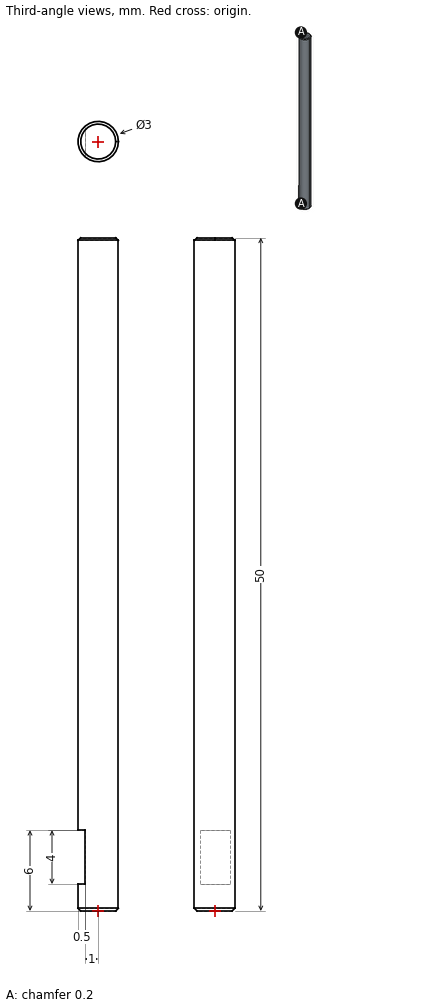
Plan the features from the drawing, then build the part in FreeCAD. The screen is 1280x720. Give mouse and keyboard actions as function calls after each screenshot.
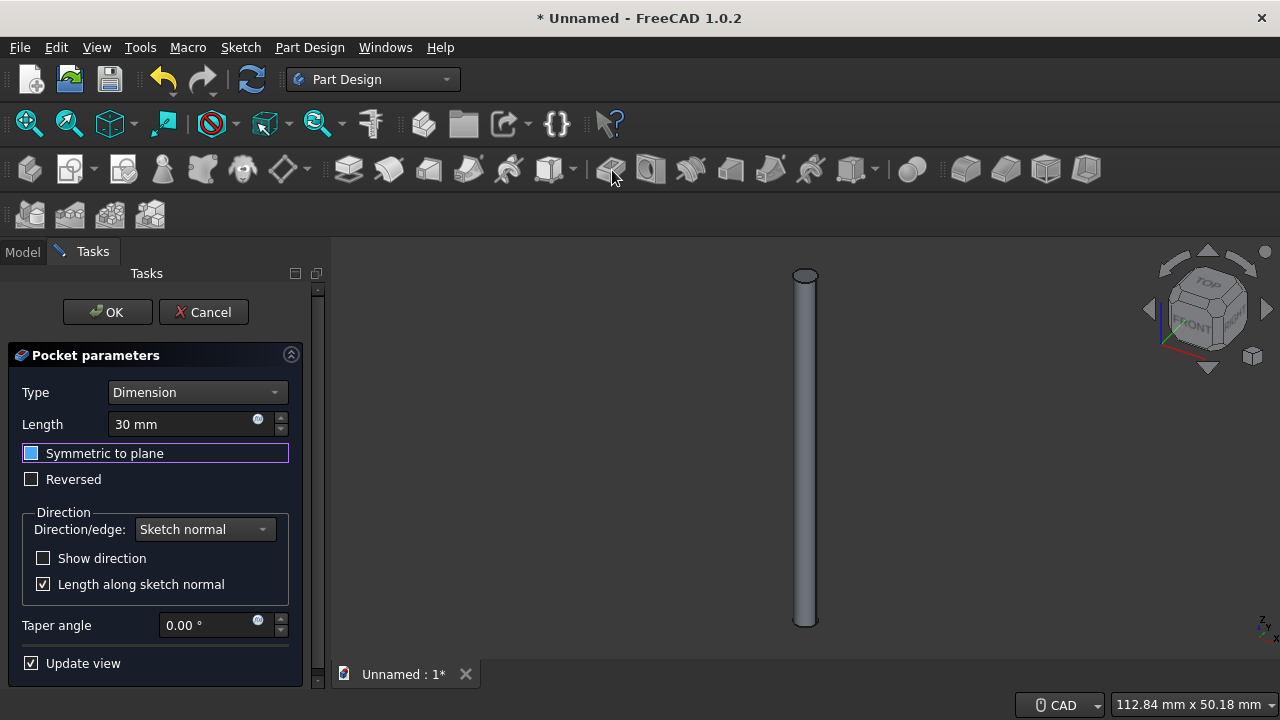
click(30, 453)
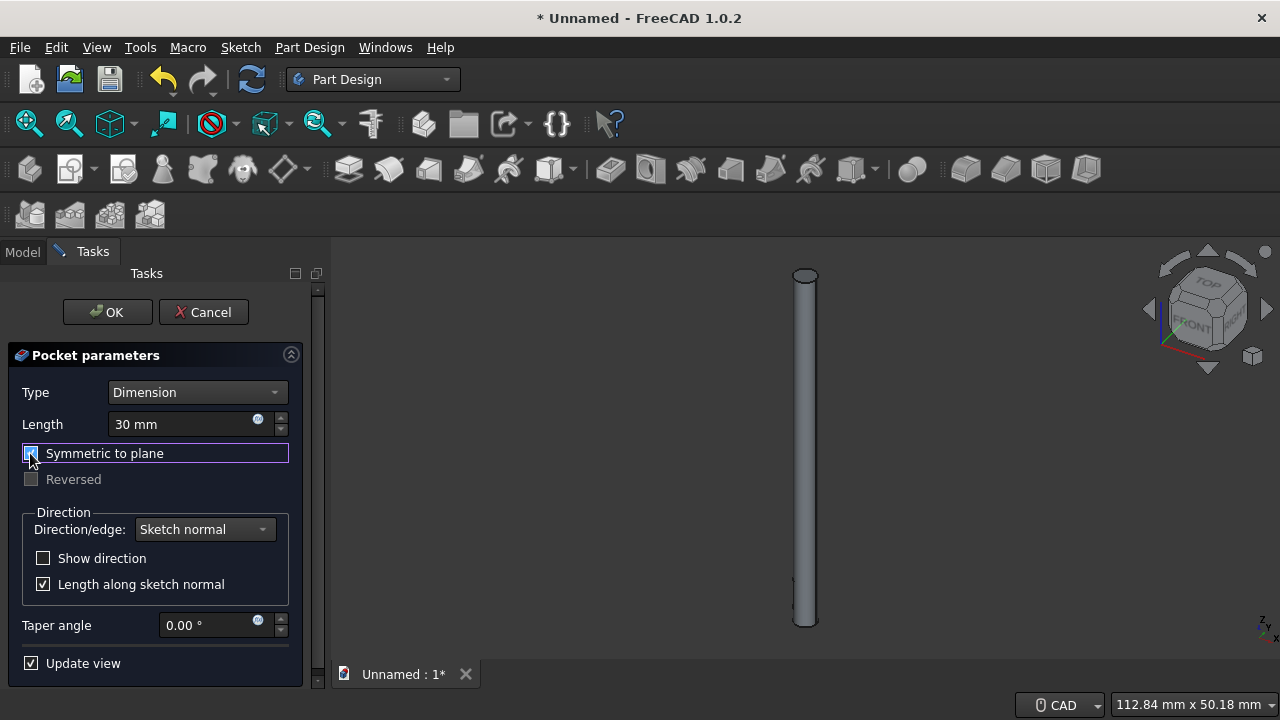
click(108, 312)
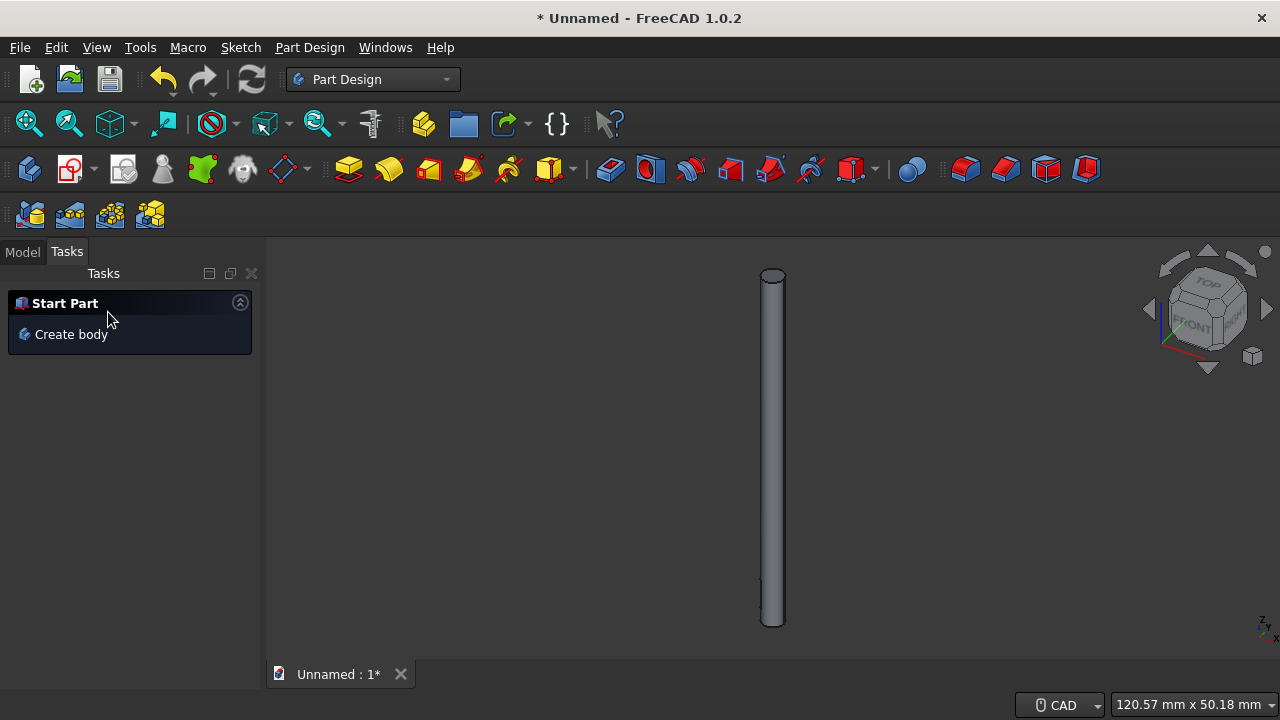
click(764, 624)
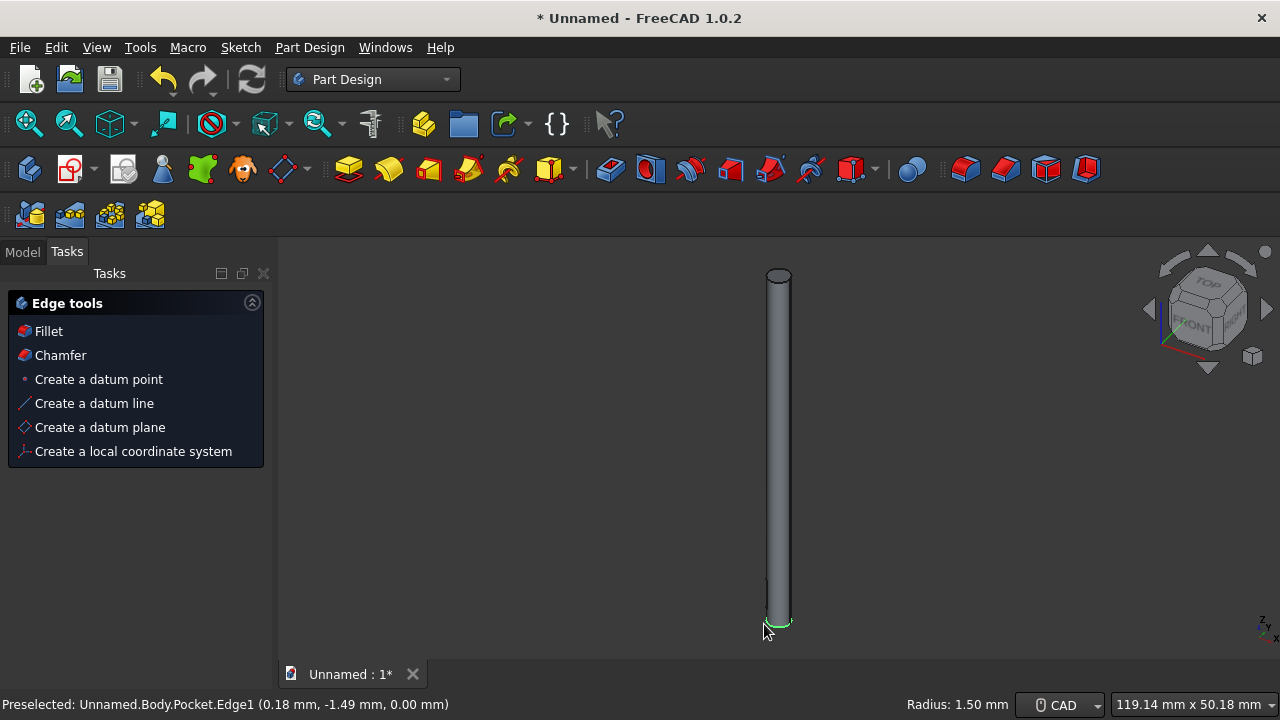
click(768, 271, ctrl)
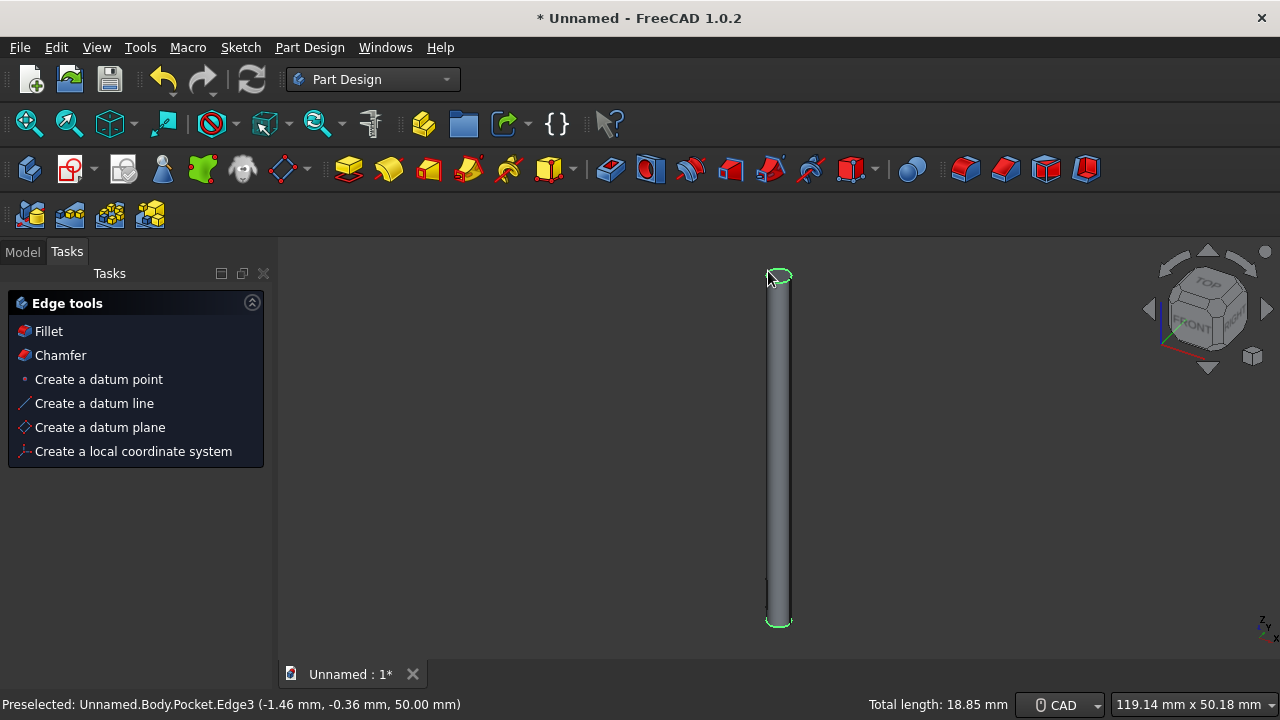
click(1006, 170)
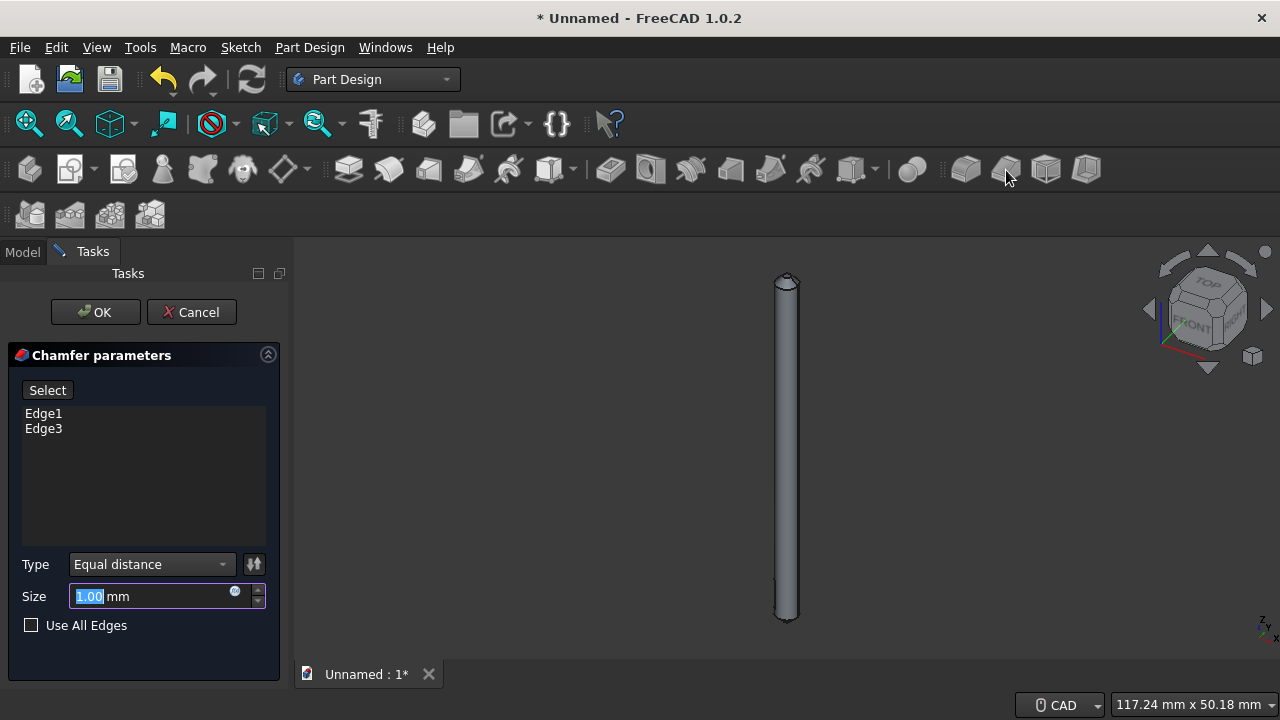
text(0.2)
key(Tab)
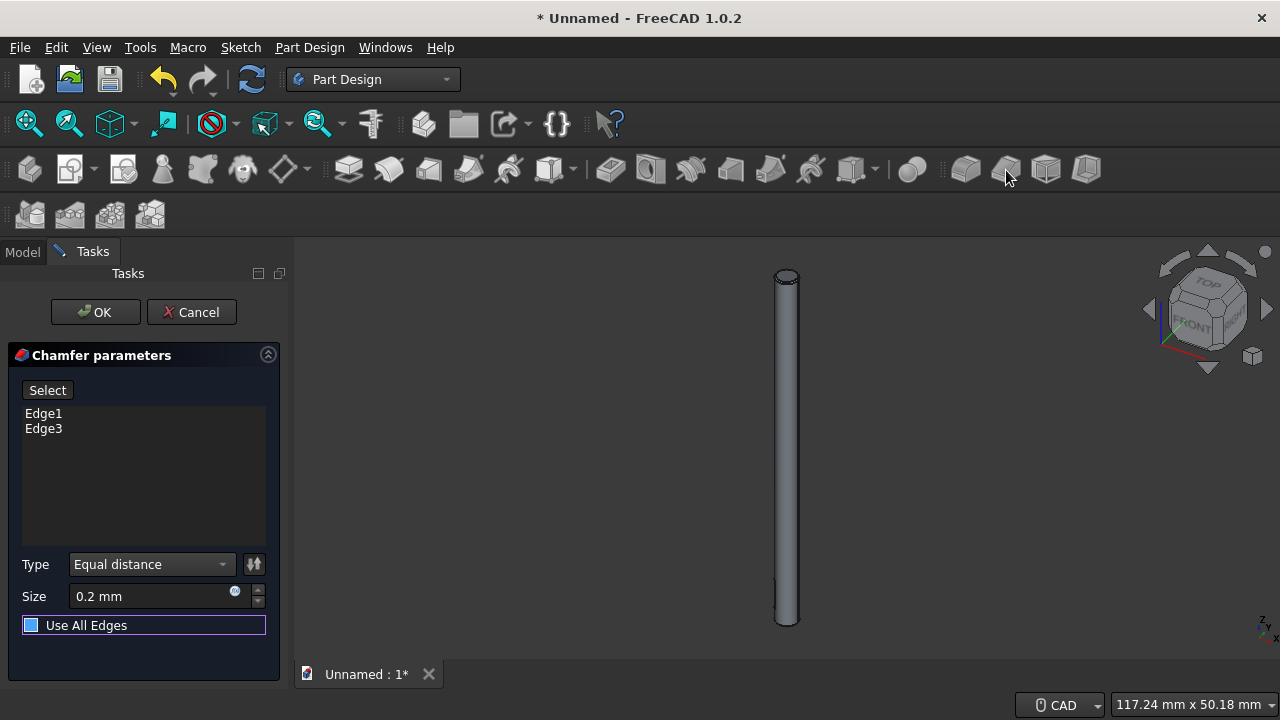
click(96, 312)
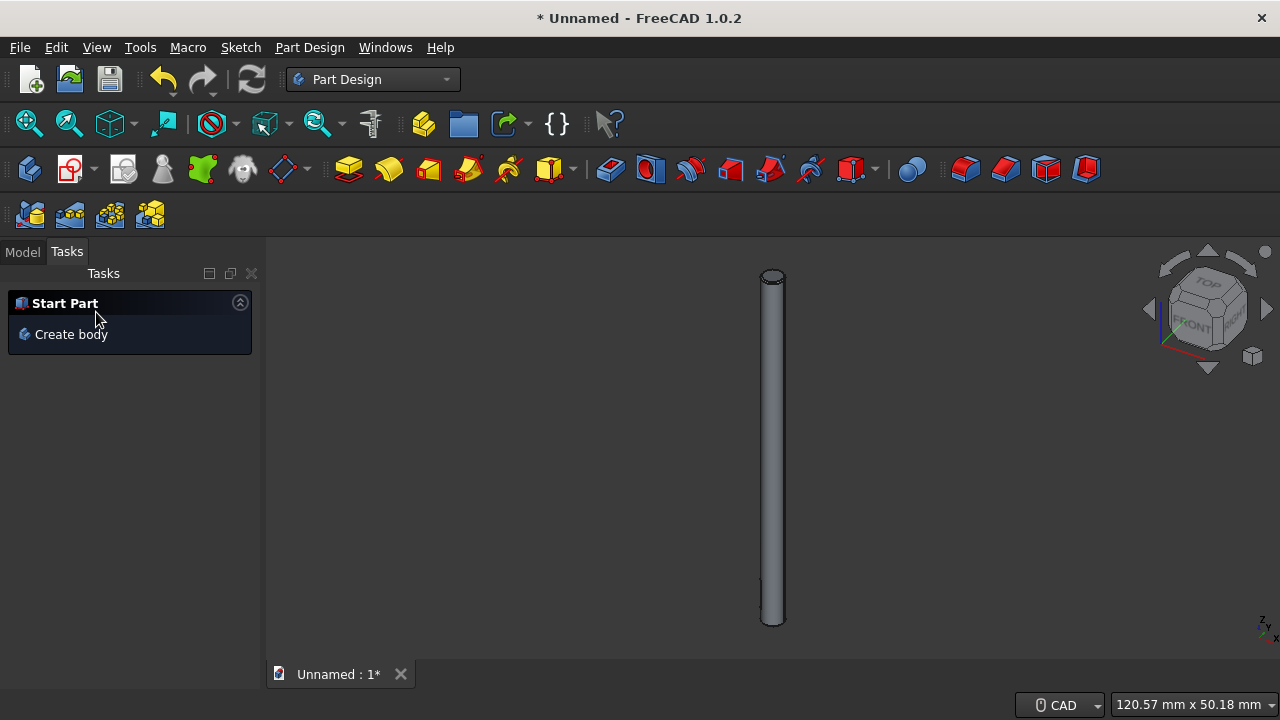
key(0)